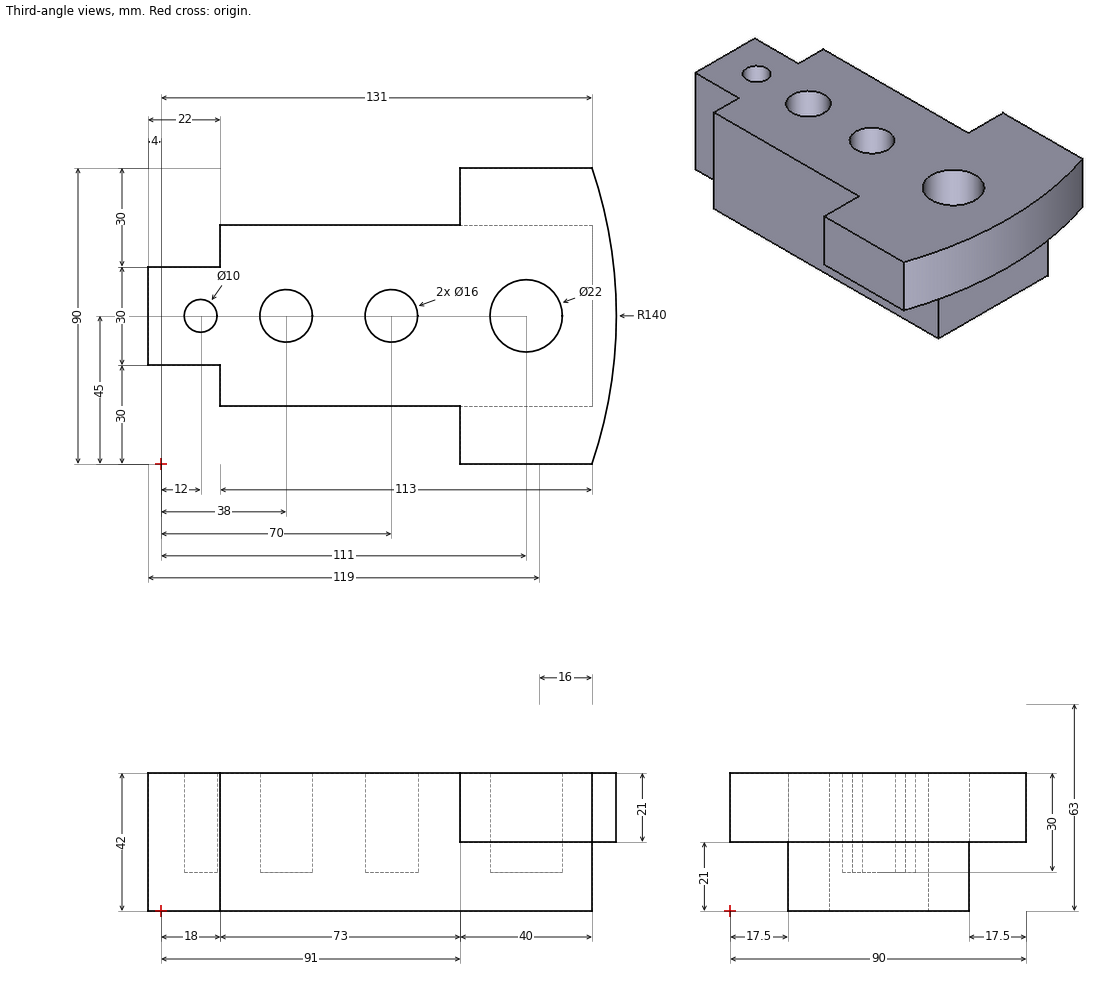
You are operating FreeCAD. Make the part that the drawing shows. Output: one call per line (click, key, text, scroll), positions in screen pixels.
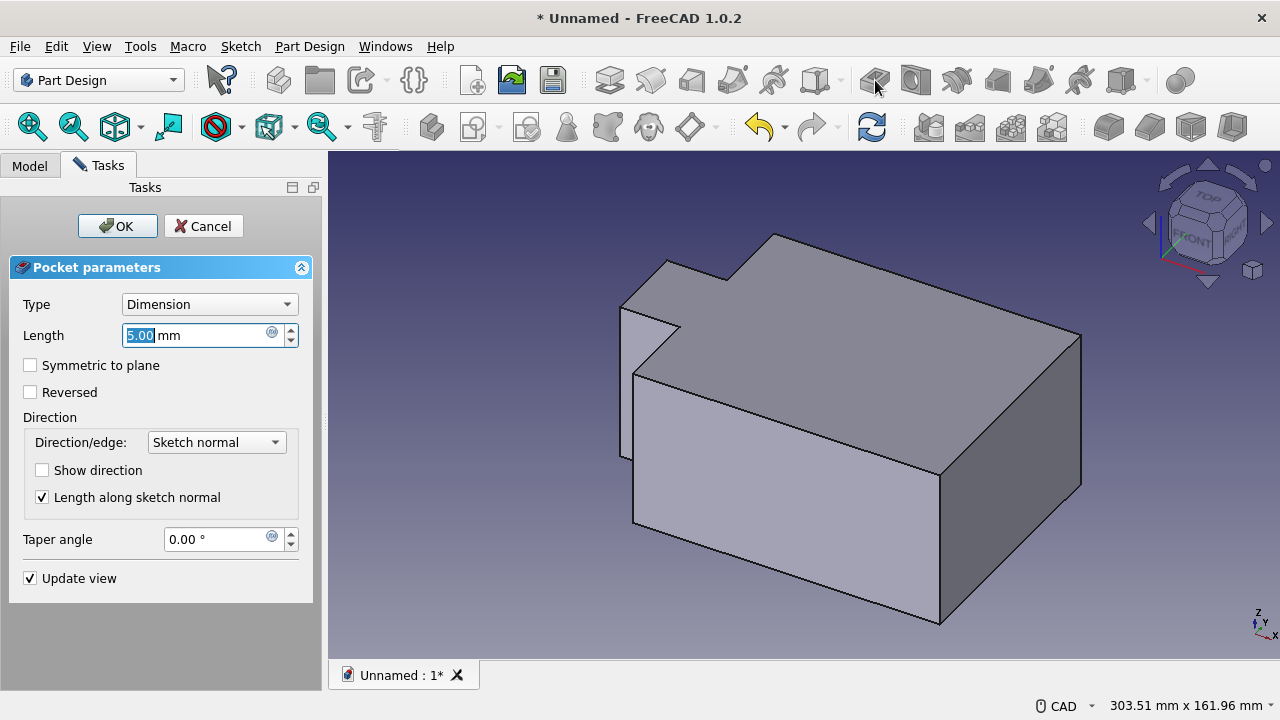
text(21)
key(Tab)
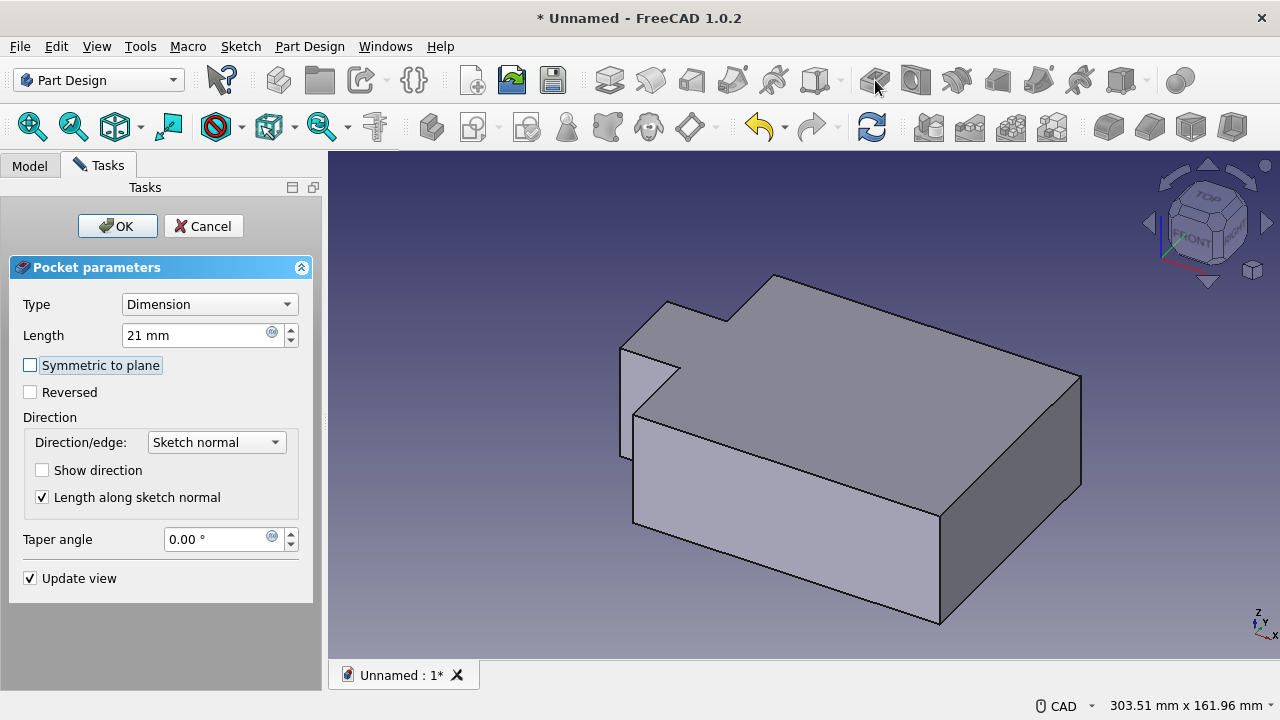
click(118, 226)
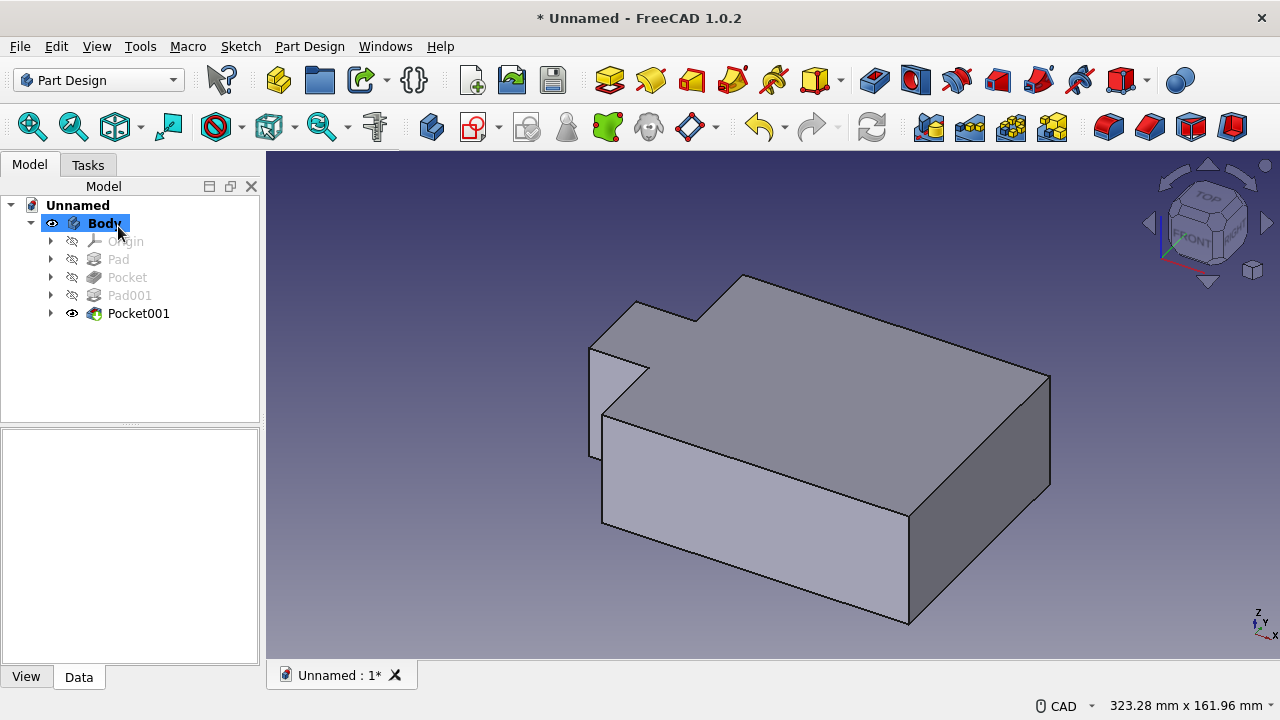
click(848, 402)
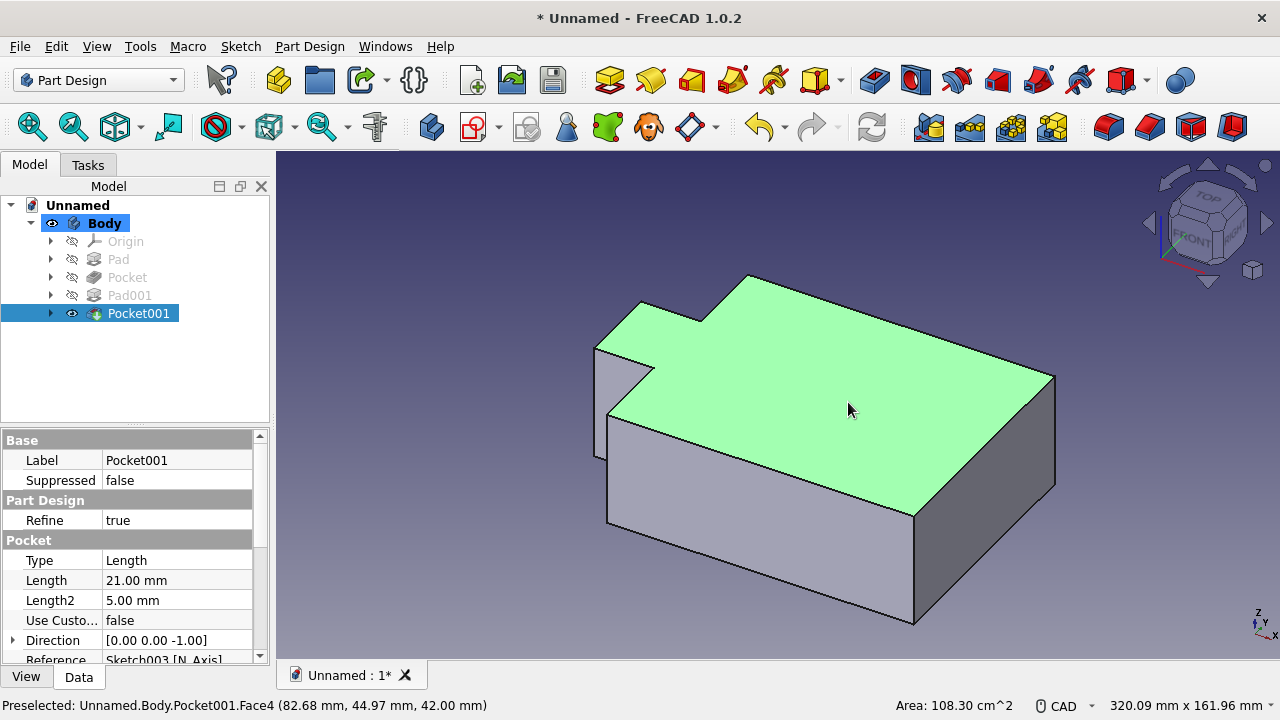
click(472, 128)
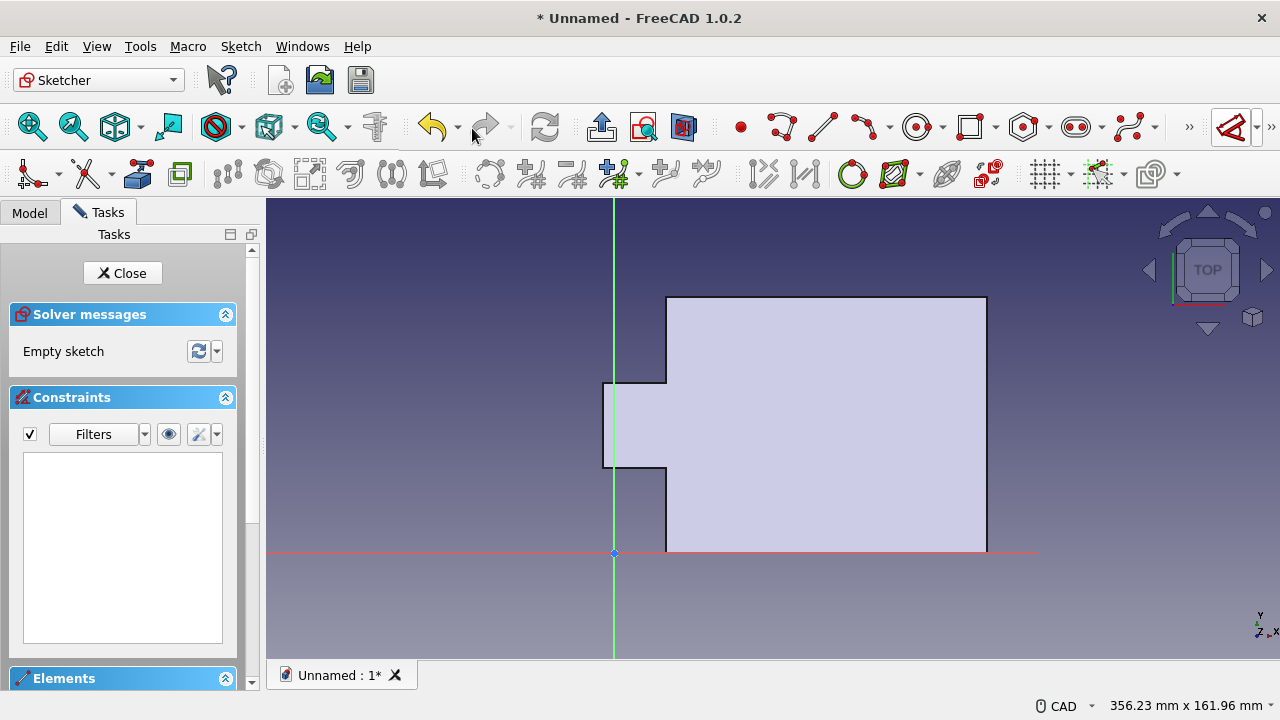
click(823, 128)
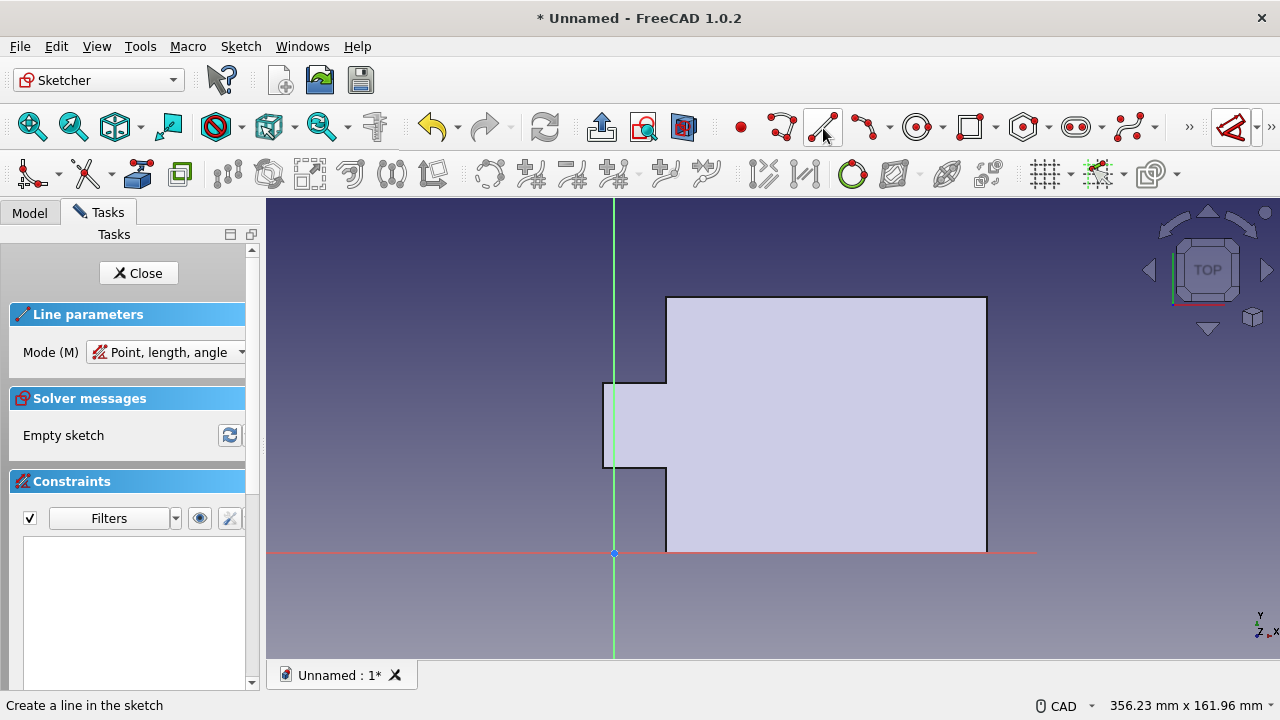
click(987, 297)
click(987, 553)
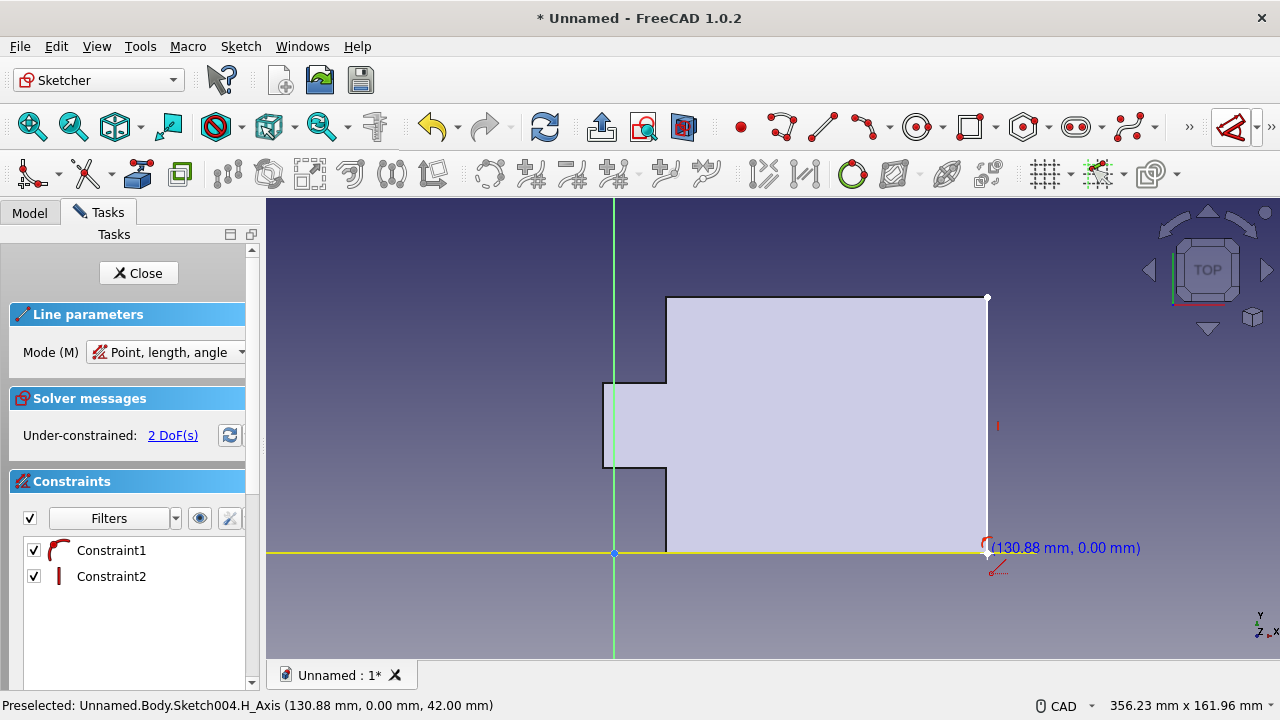
click(864, 128)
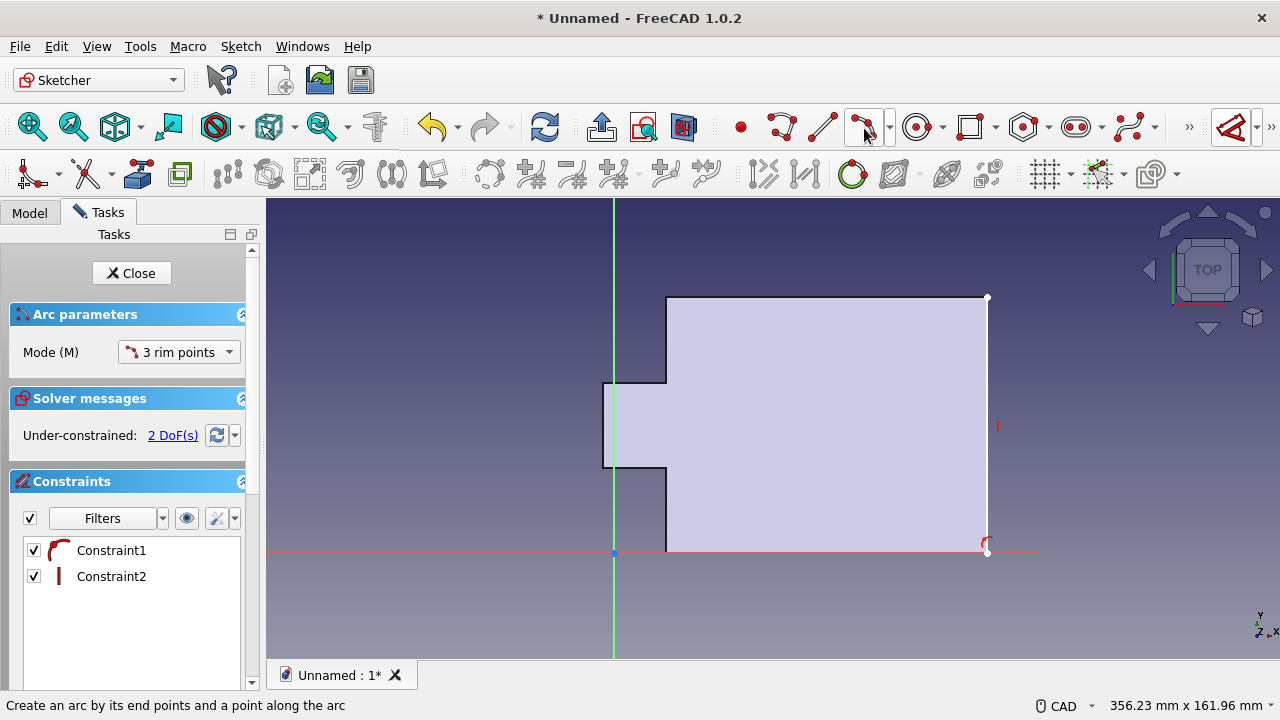
click(987, 553)
click(987, 298)
click(1008, 425)
key(Escape)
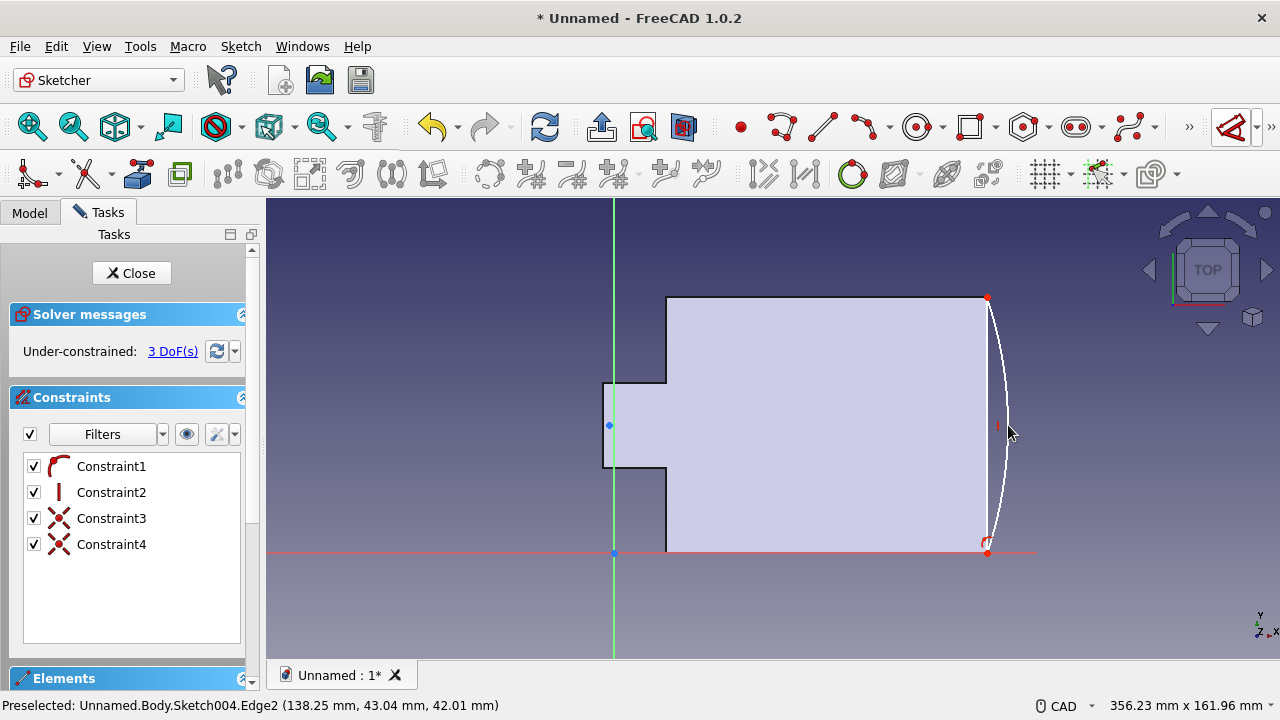
click(1005, 478)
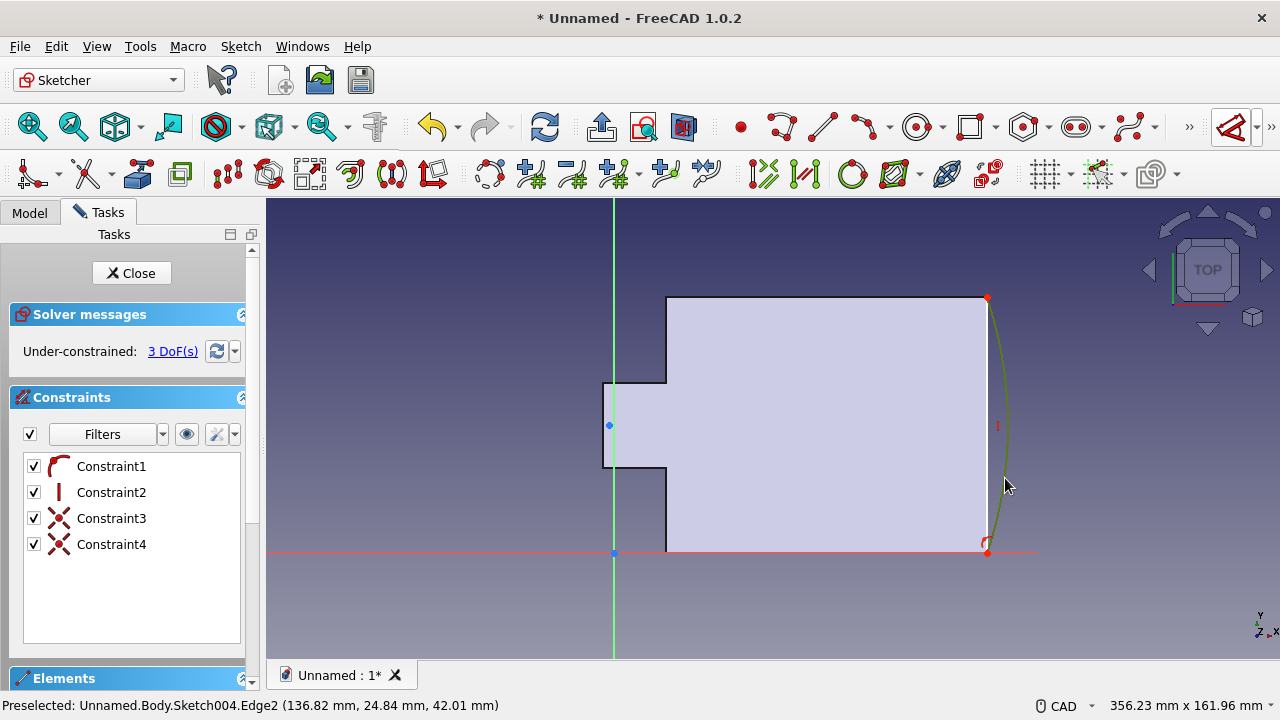
key(k)
key(r)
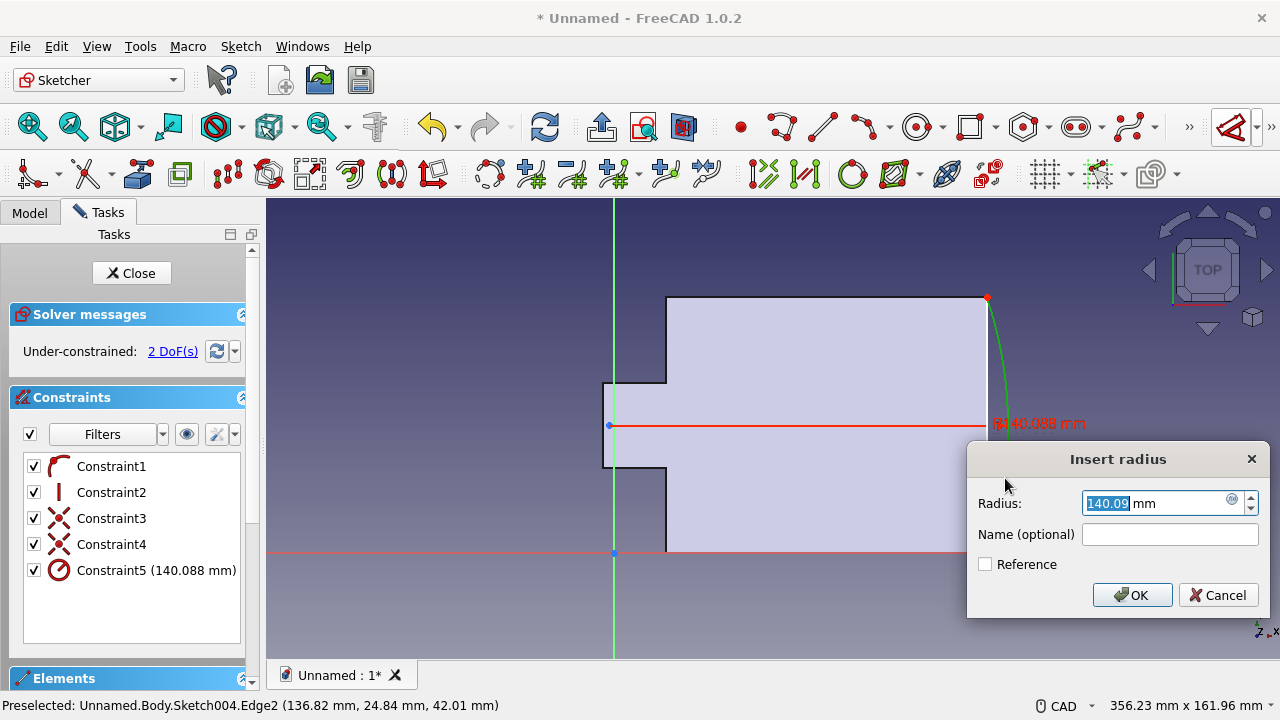
text(140)
key(Return)